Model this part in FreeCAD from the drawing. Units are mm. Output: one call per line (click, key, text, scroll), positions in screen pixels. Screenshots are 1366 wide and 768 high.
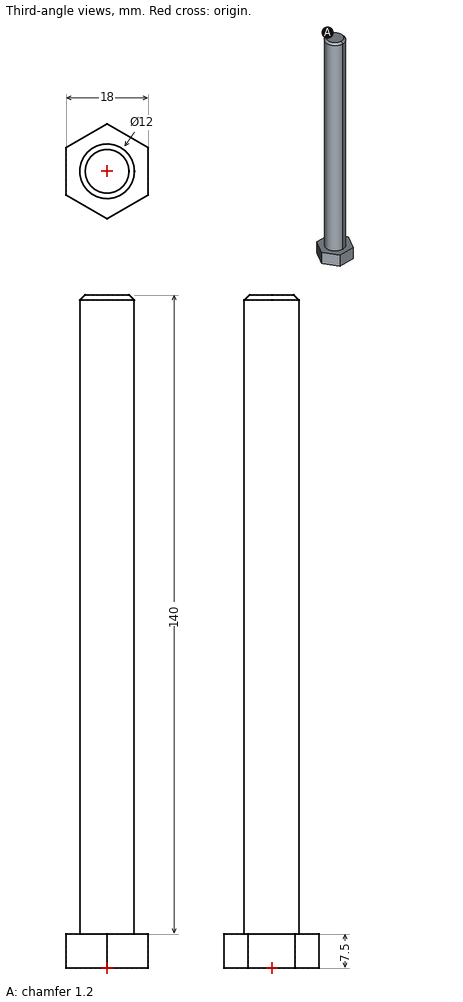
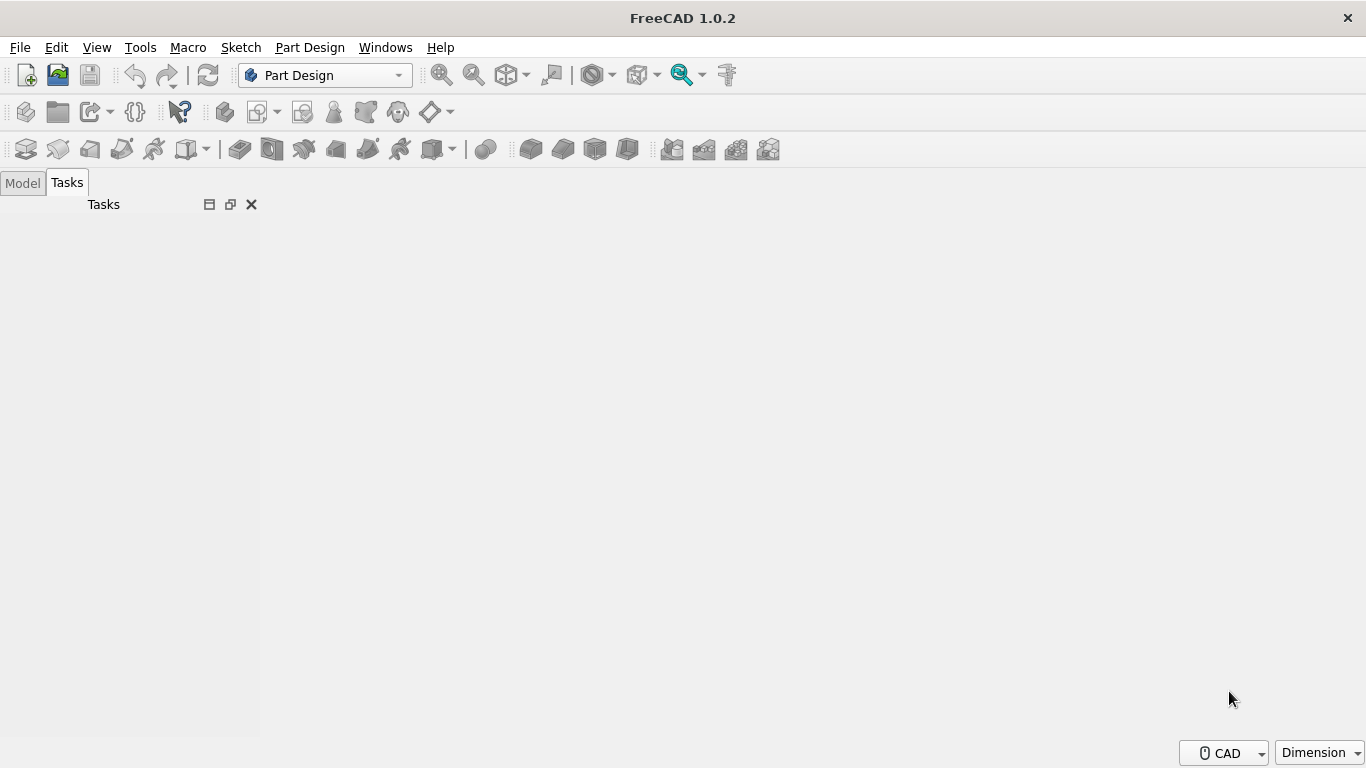
key(ctrl+n)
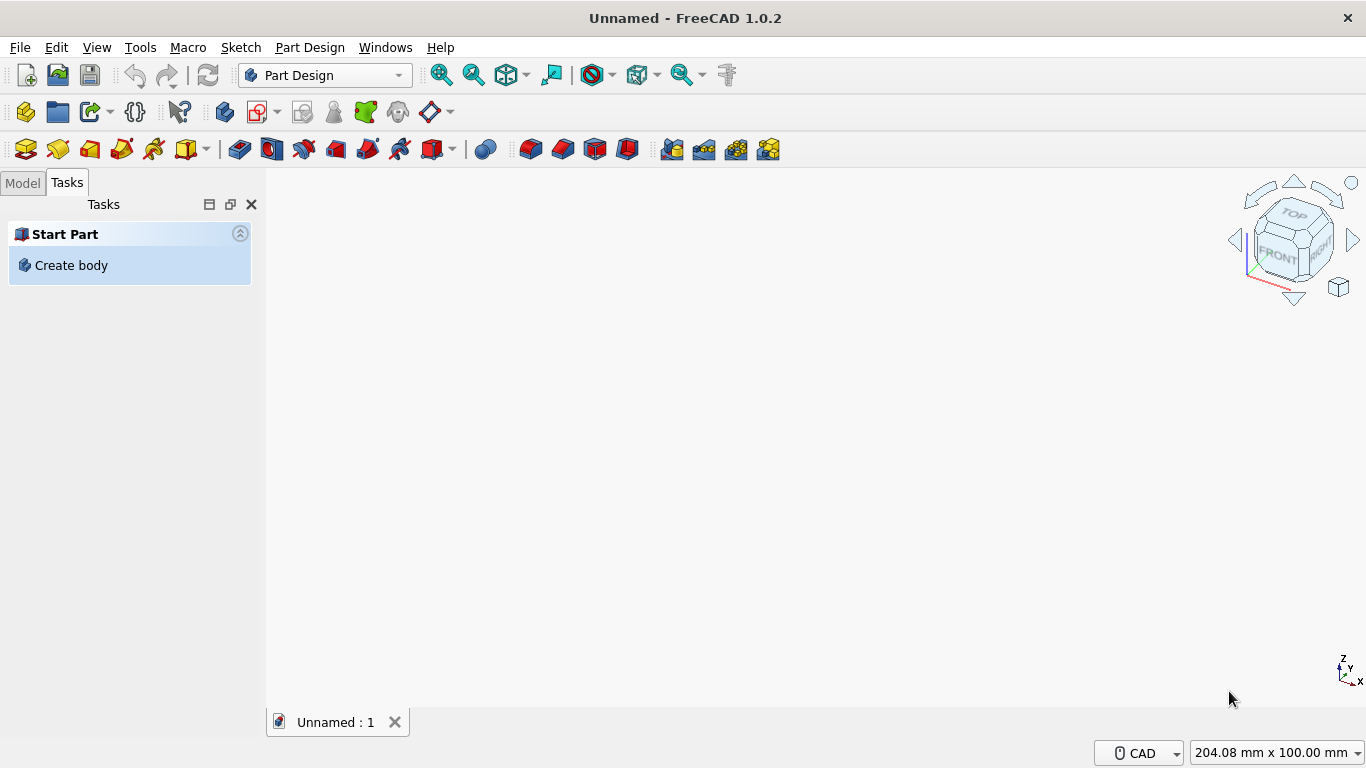
click(258, 112)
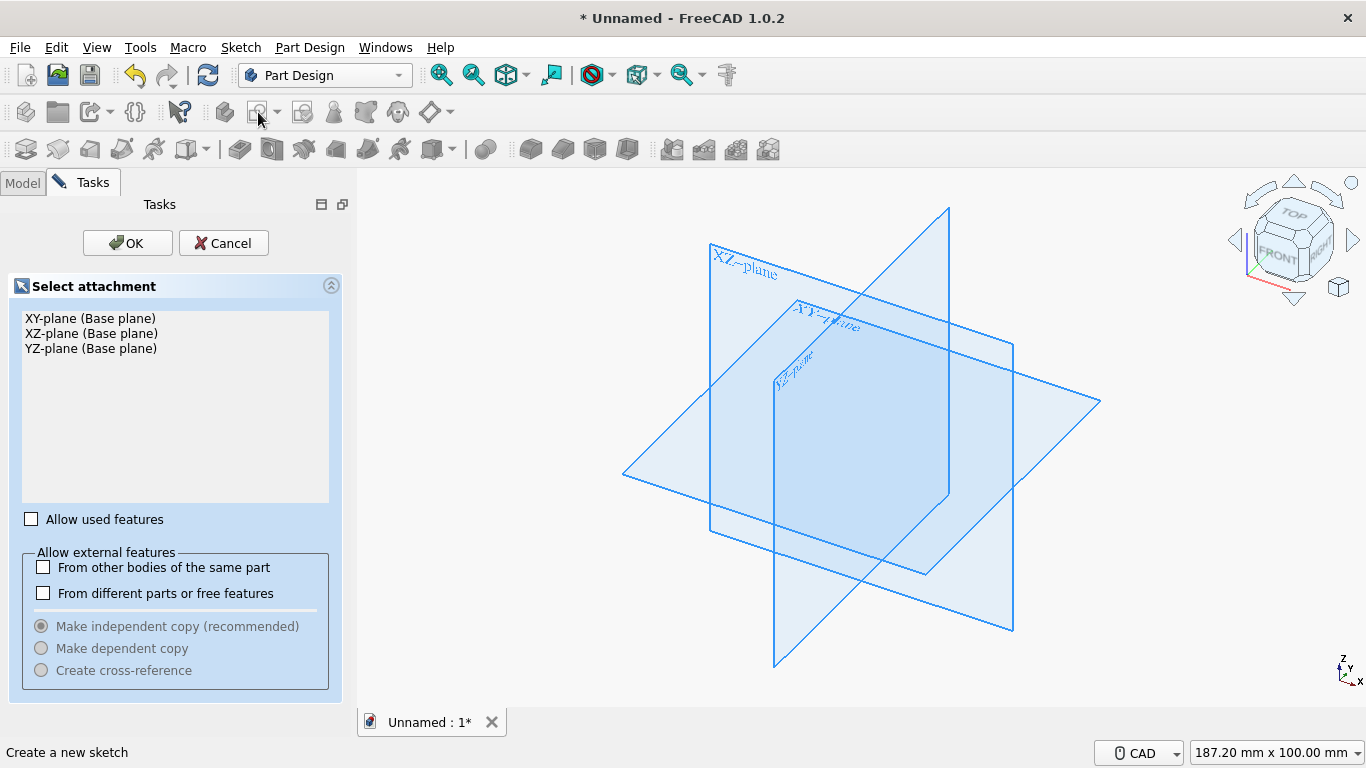
click(82, 318)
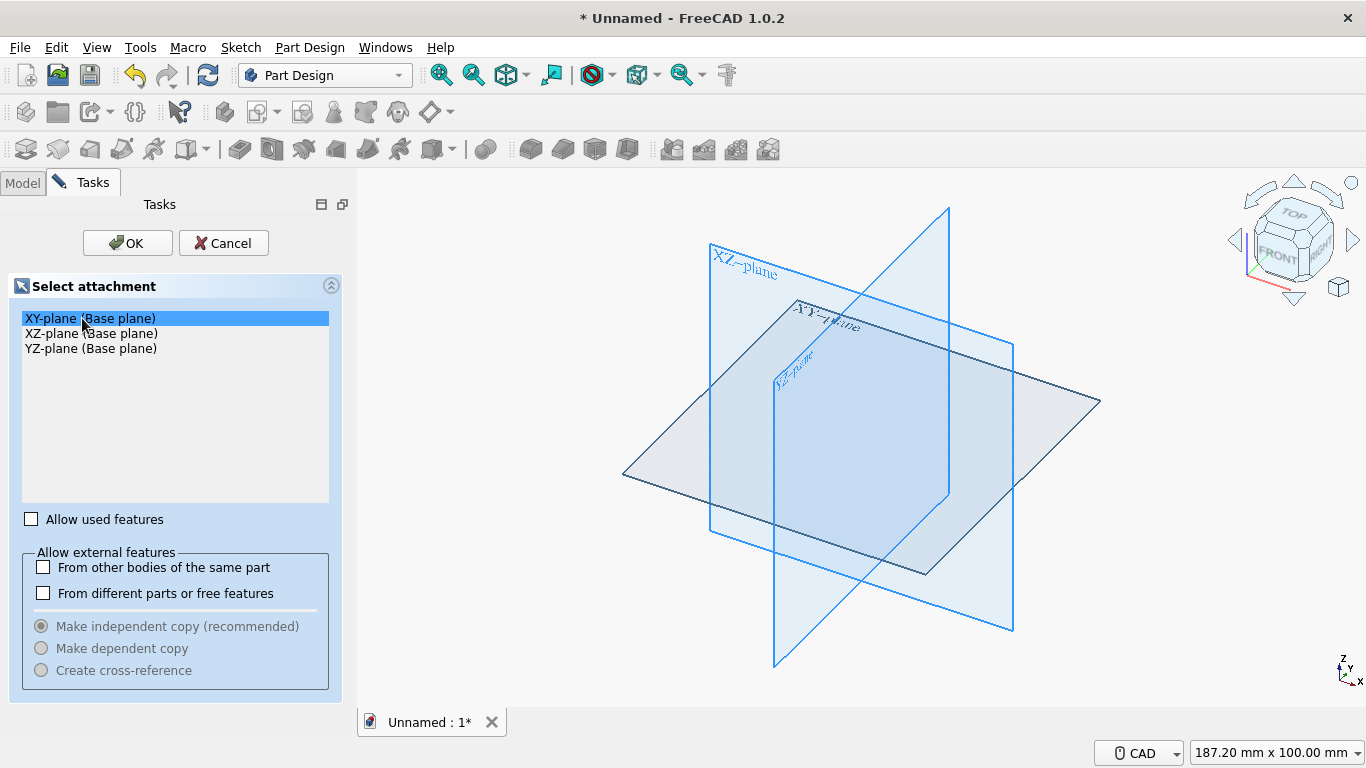
click(128, 243)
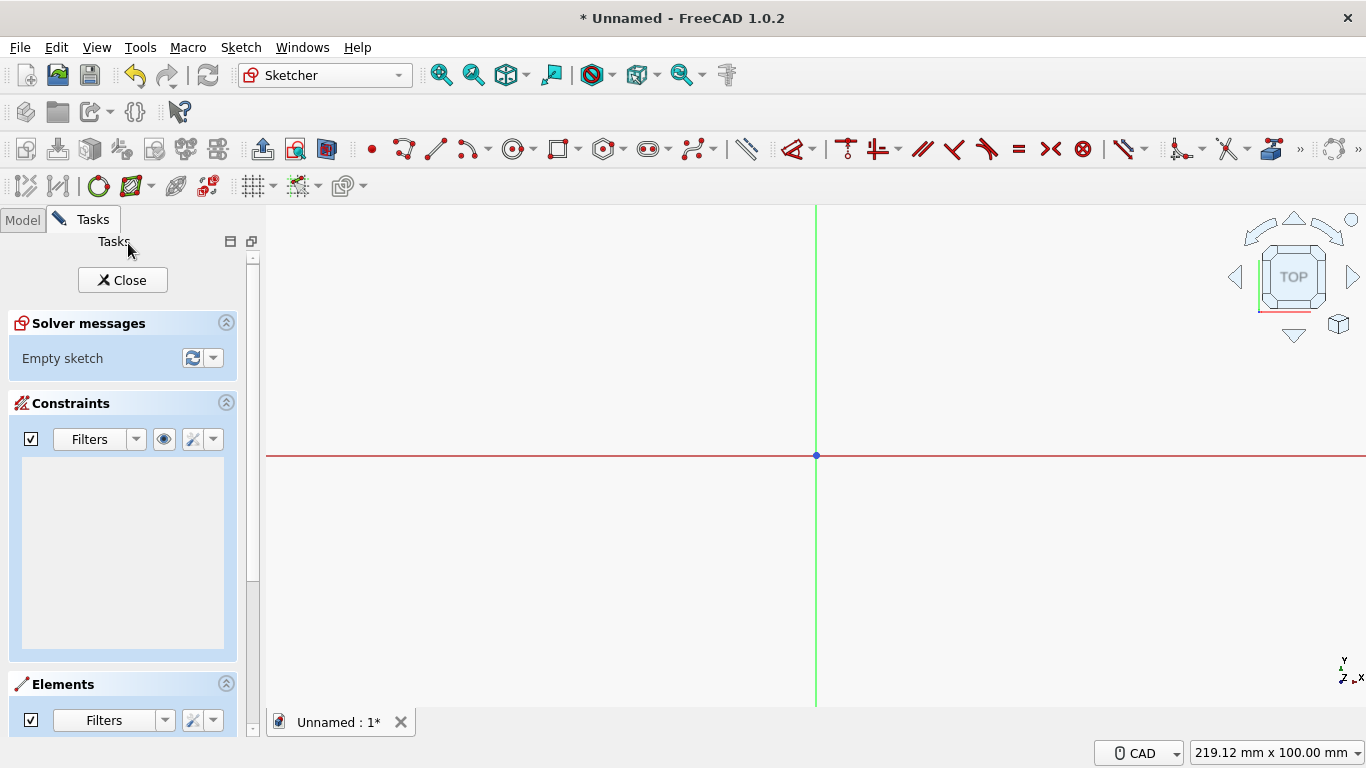
scroll(846, 456, up, 6)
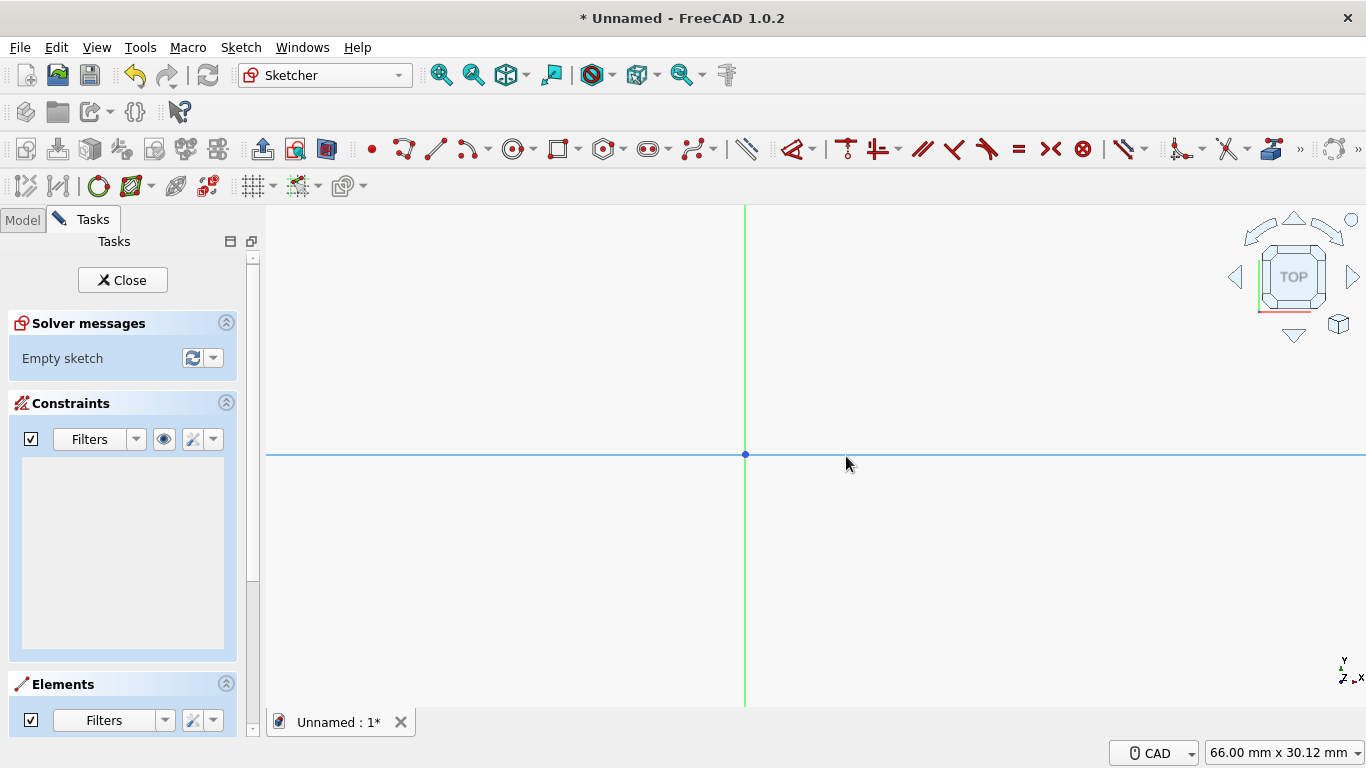
click(604, 150)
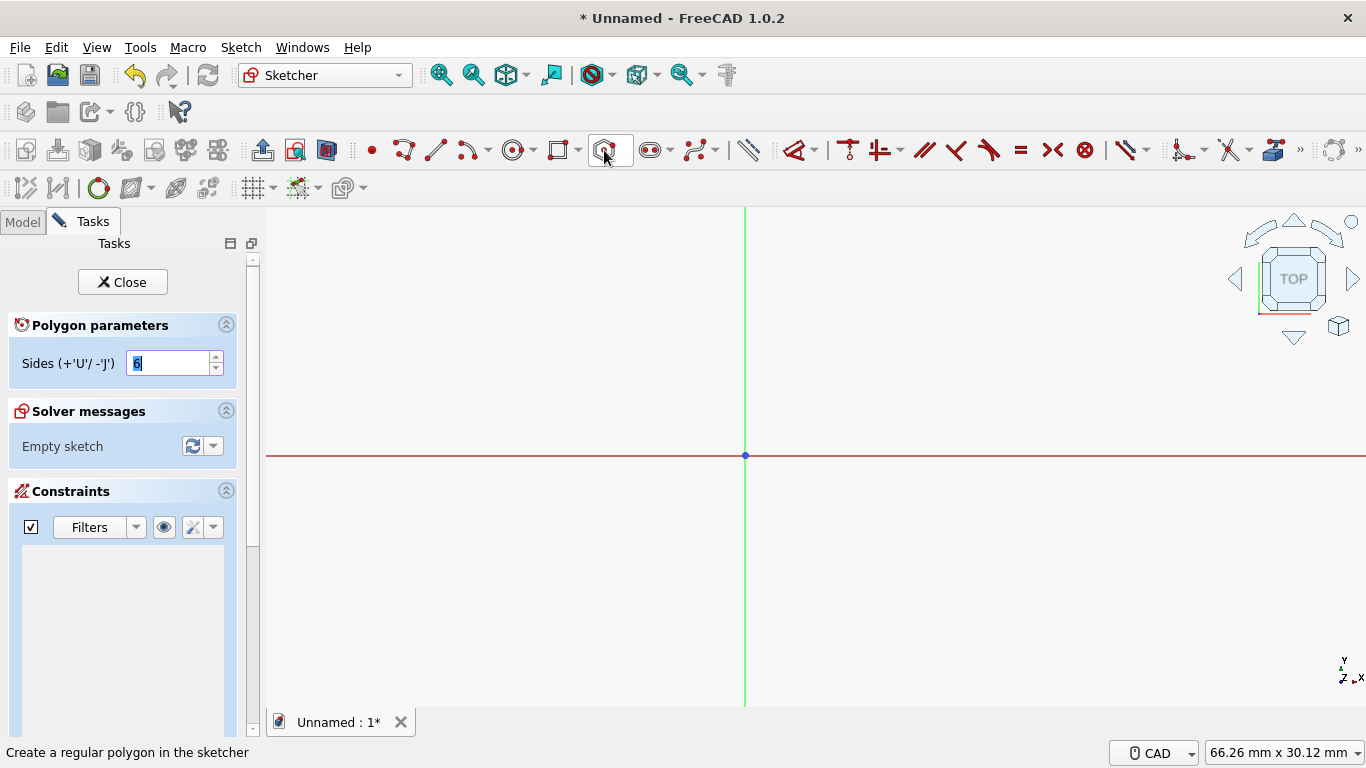
click(745, 456)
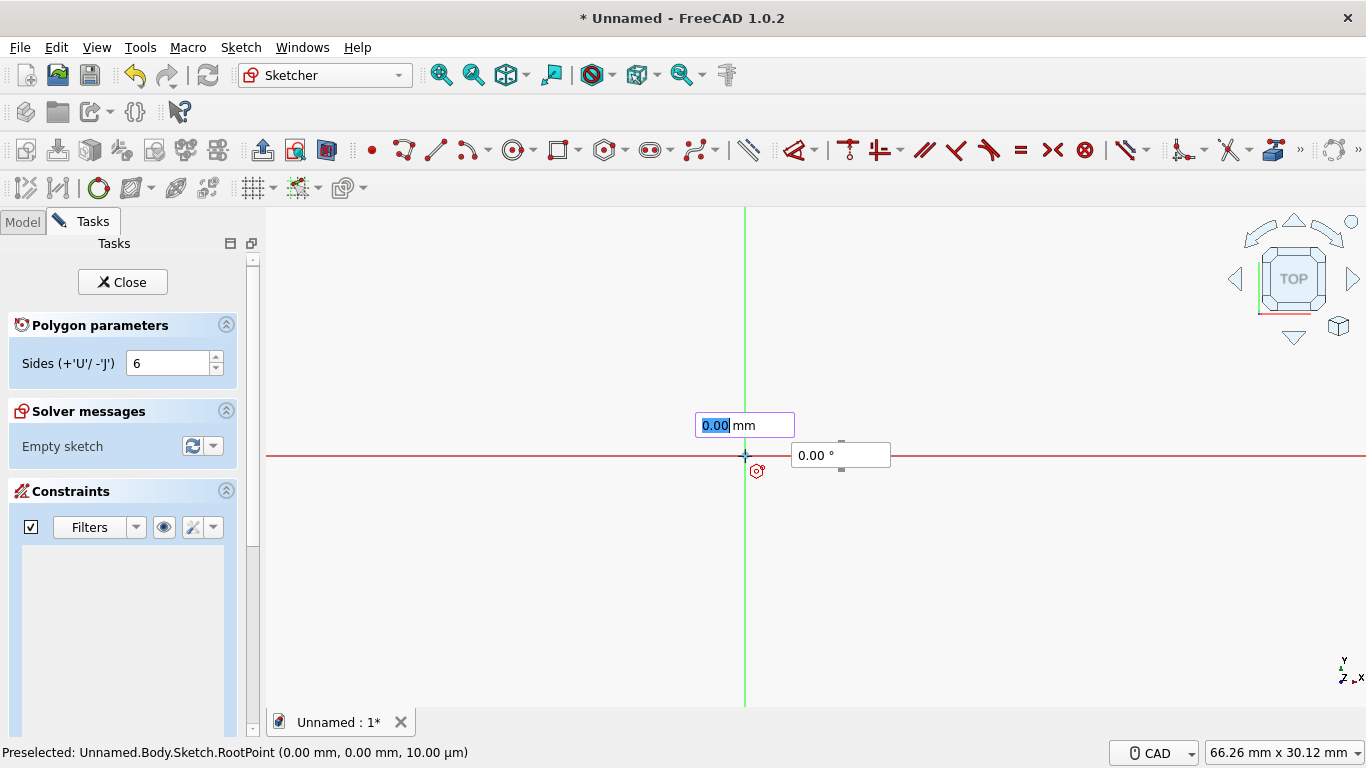
click(745, 283)
right_click(745, 283)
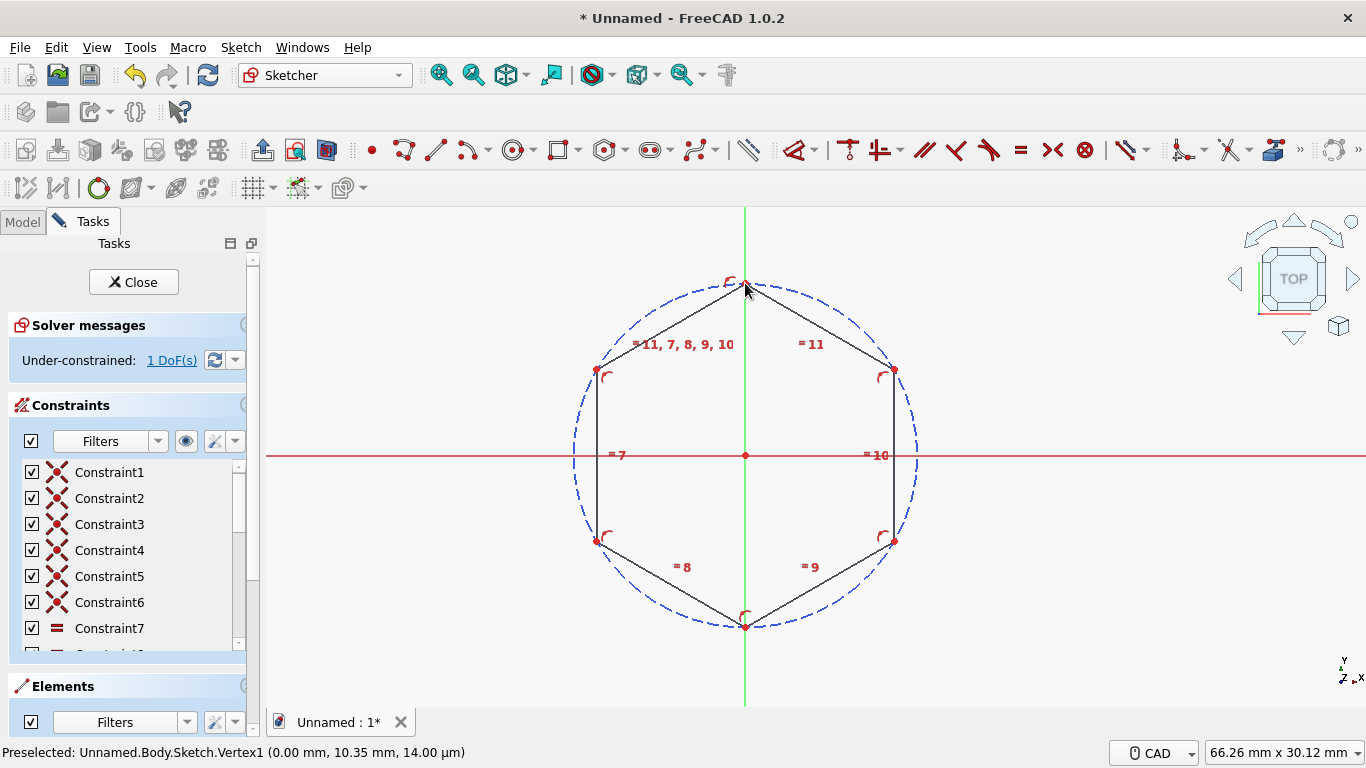
click(597, 370)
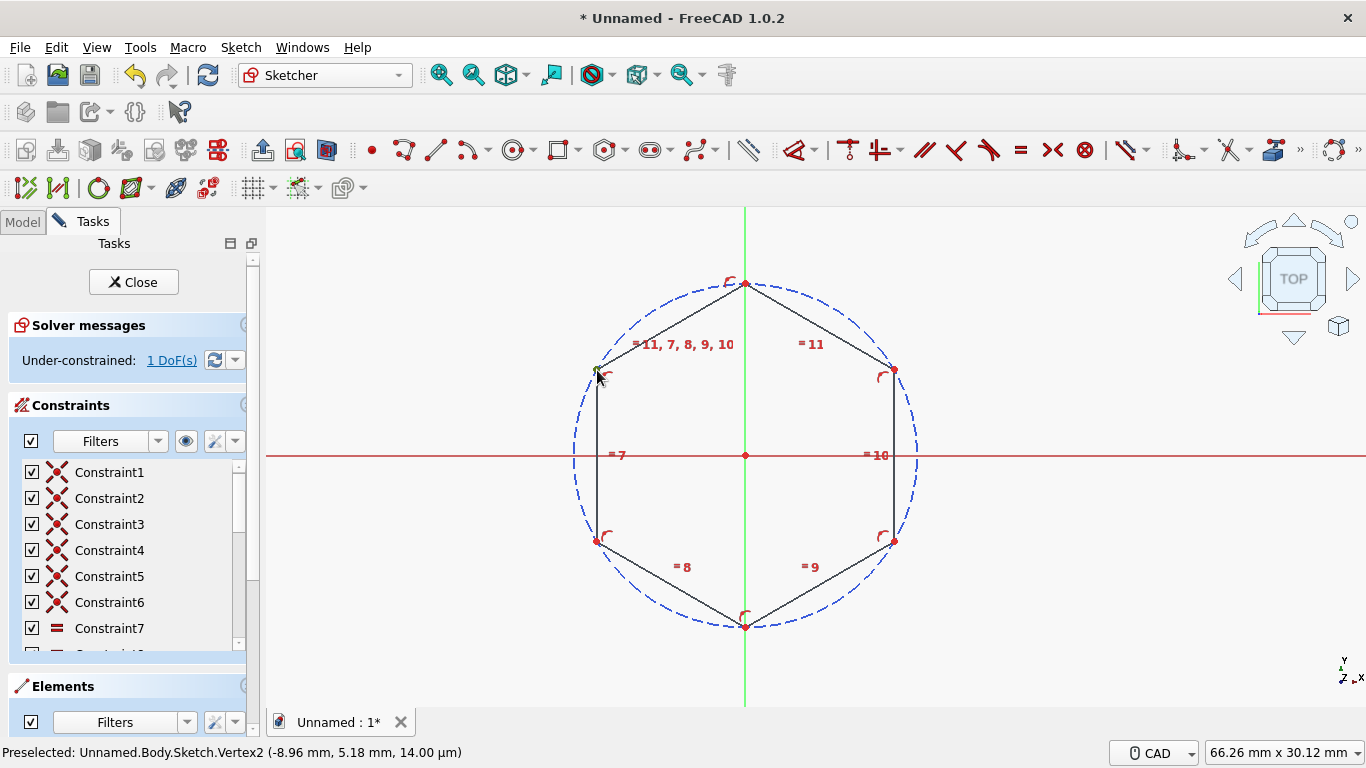
click(894, 542)